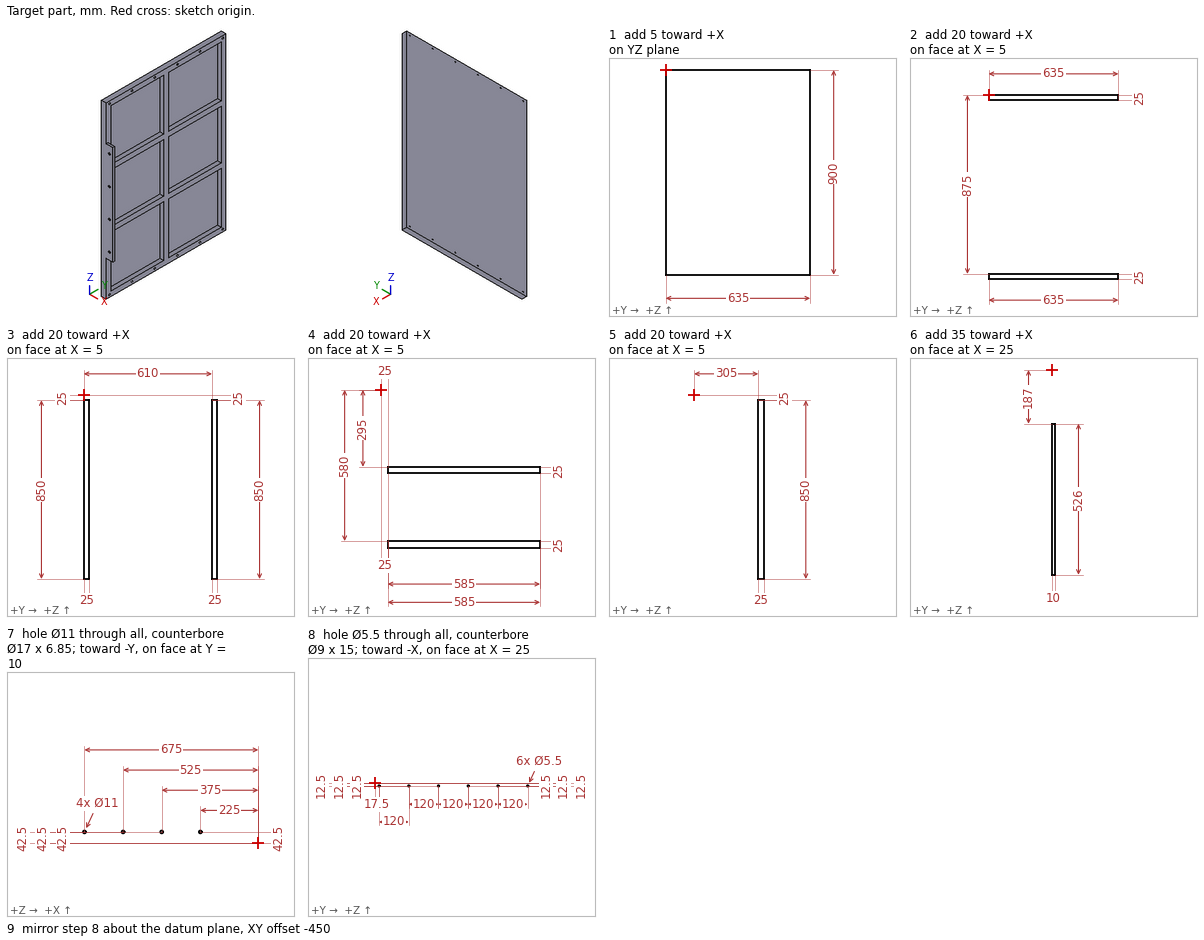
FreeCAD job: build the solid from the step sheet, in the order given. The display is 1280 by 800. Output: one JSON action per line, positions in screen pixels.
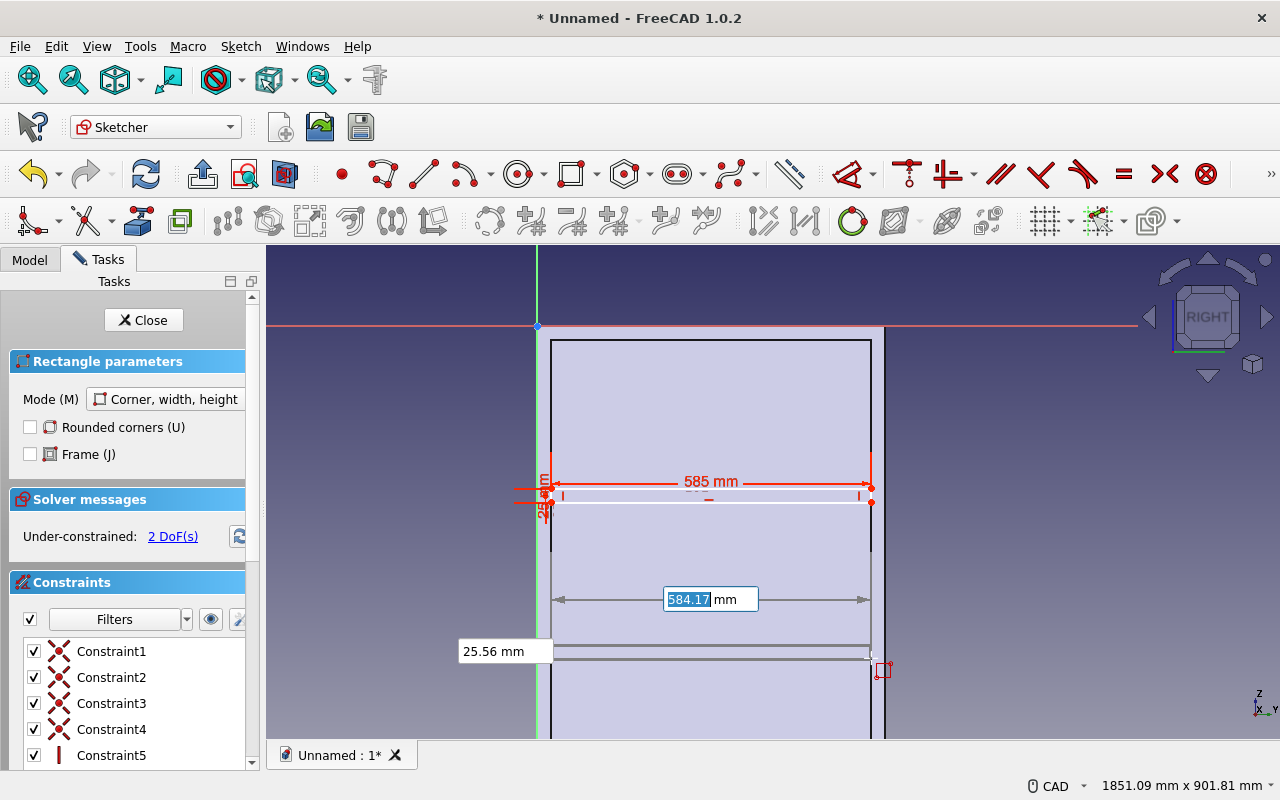
{"action": "type", "text": "585"}
{"action": "key", "text": "Tab"}
{"action": "type", "text": "25"}
{"action": "key", "text": "Return"}
{"action": "key", "text": "Escape"}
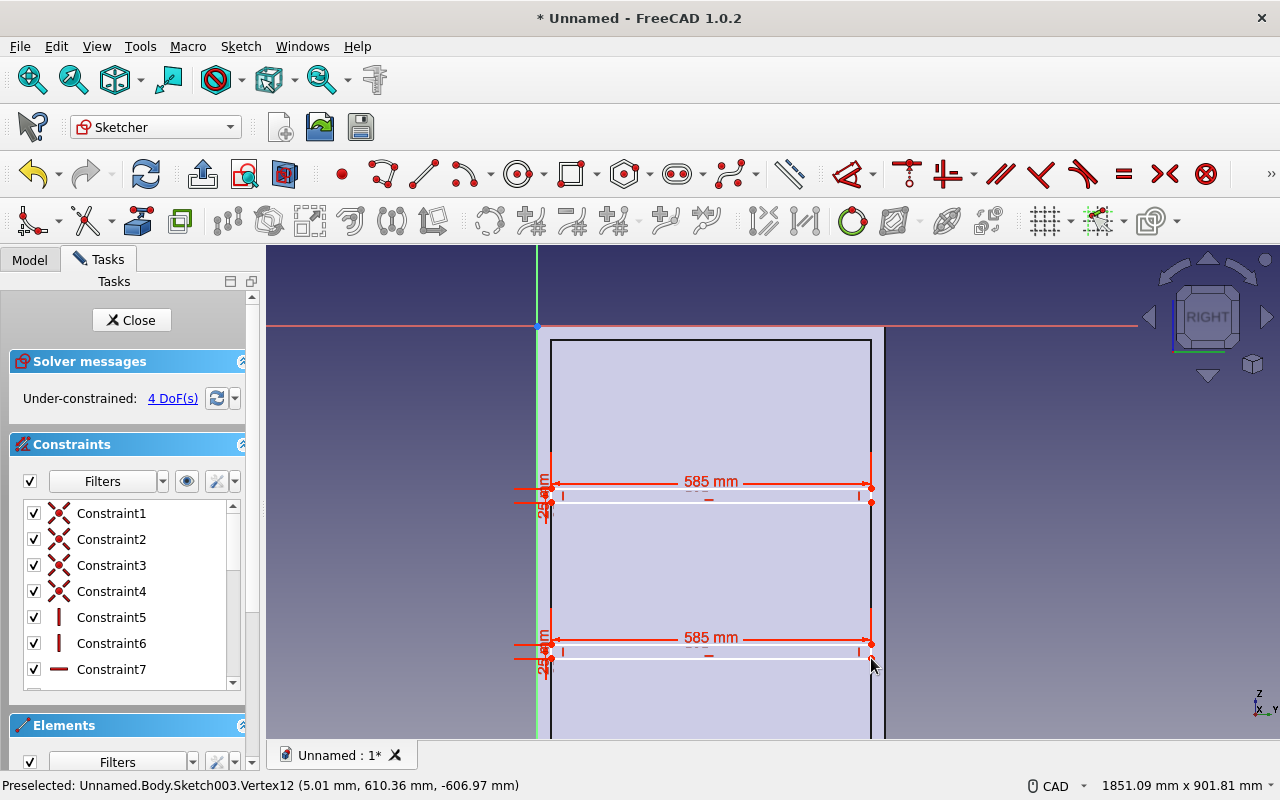
{"action": "key", "text": "d"}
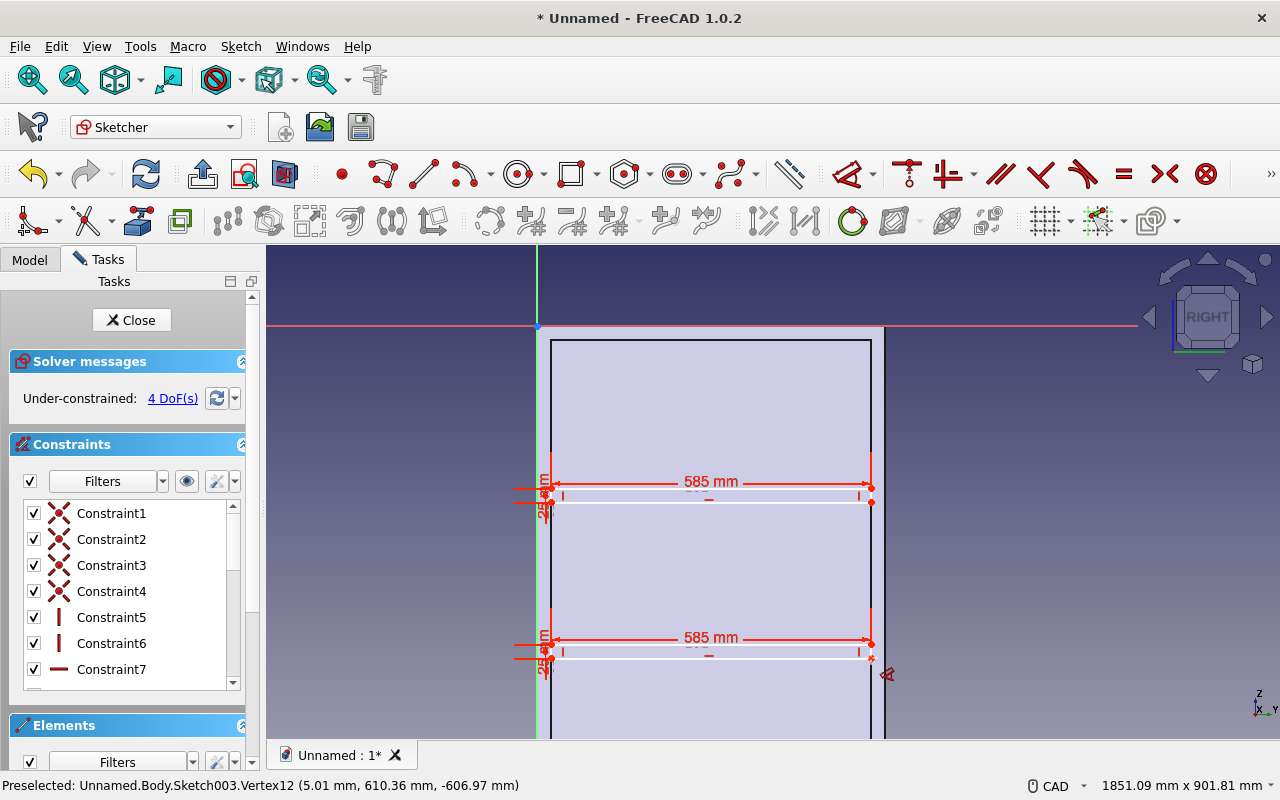
{"action": "scroll", "coordinate": [551, 489], "scroll_direction": "up", "scroll_amount": 6}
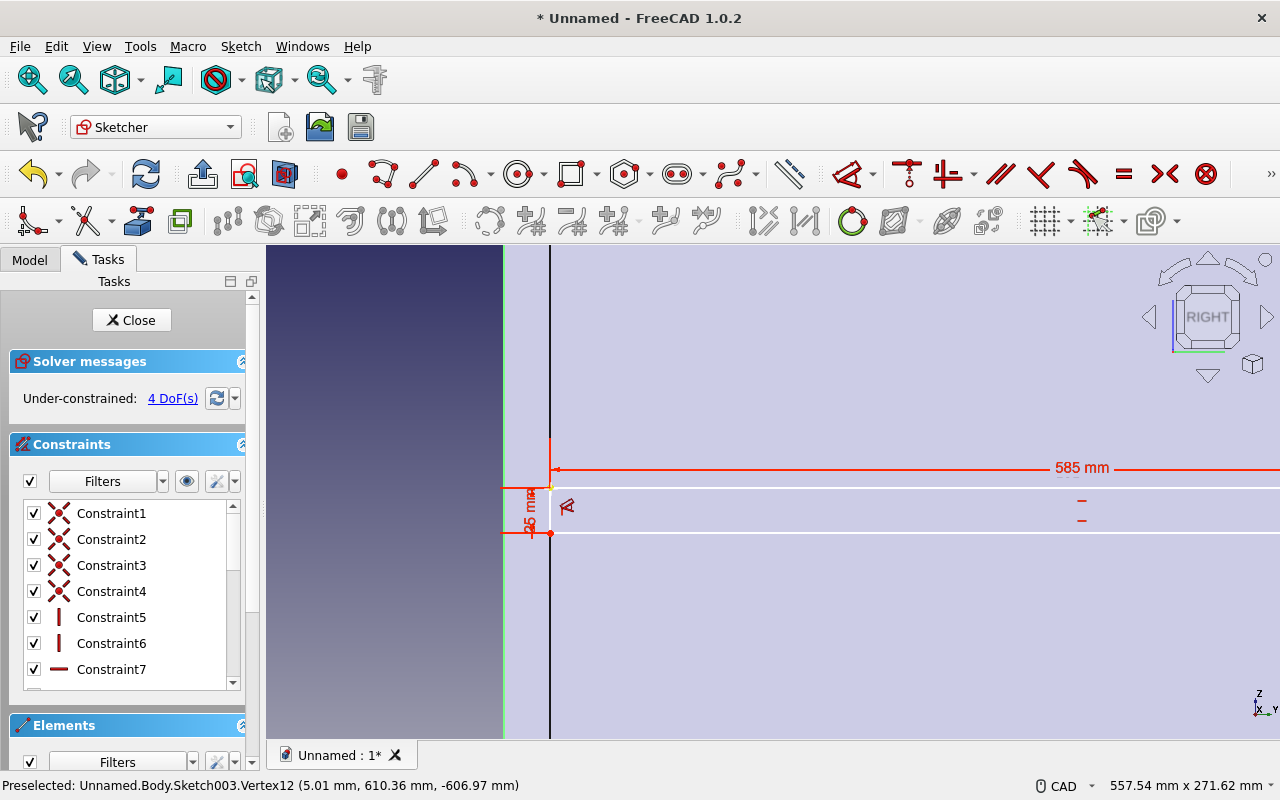
{"action": "left_click", "coordinate": [550, 488]}
{"action": "left_click", "coordinate": [527, 522]}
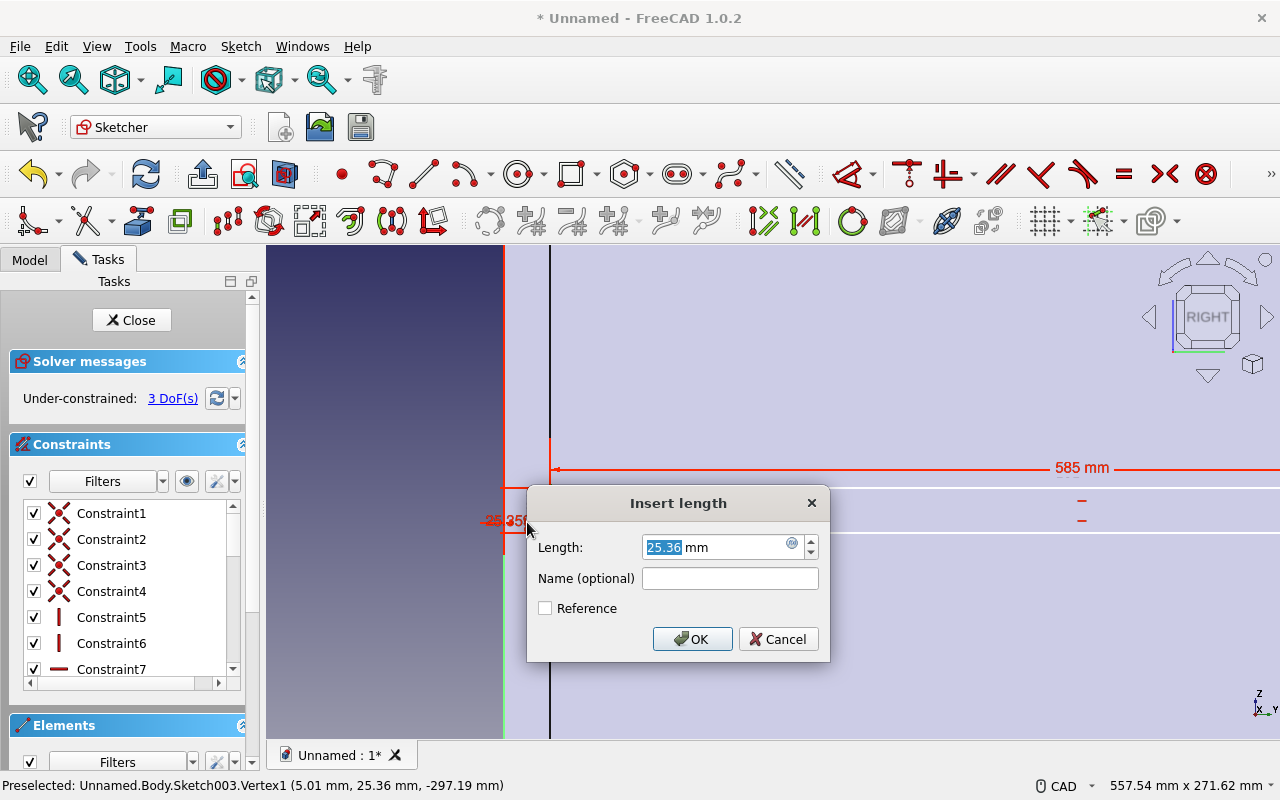
{"action": "type", "text": "25"}
{"action": "key", "text": "Return"}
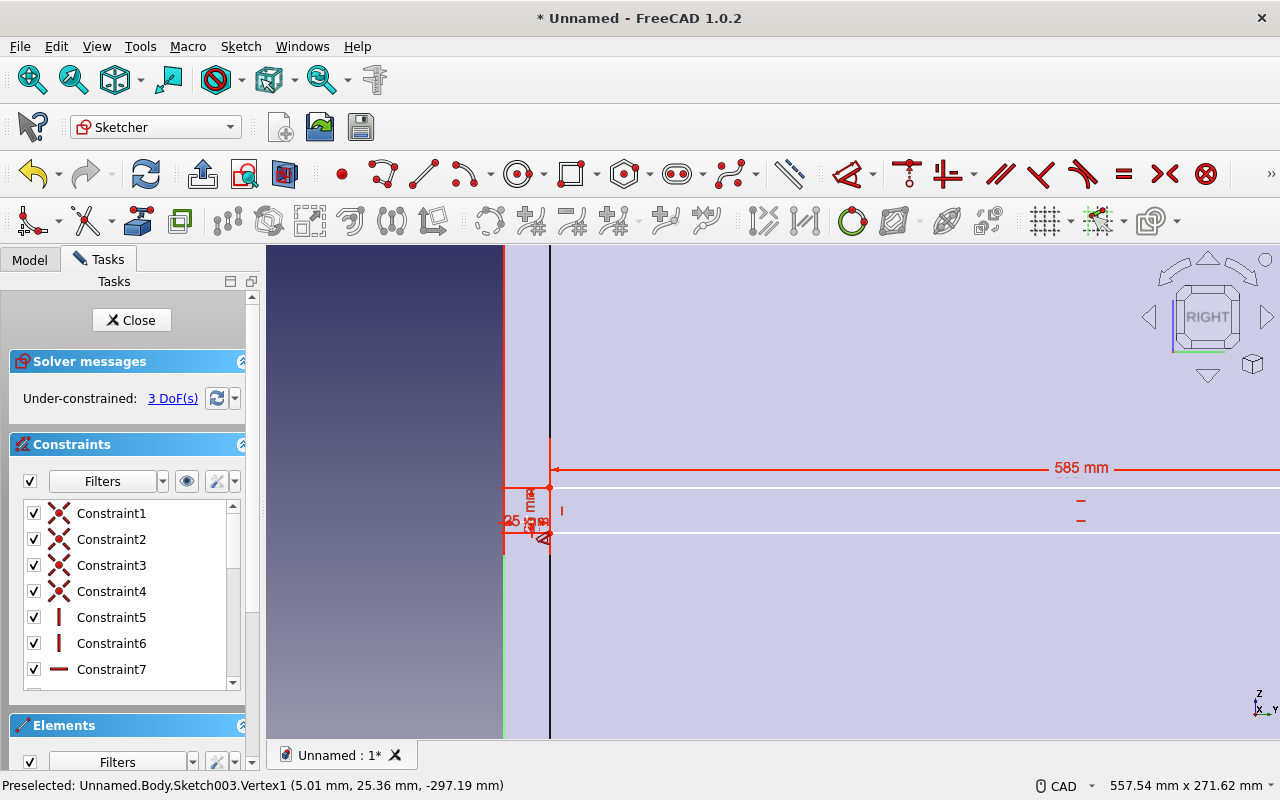
{"action": "scroll", "coordinate": [552, 490], "scroll_direction": "down", "scroll_amount": 6}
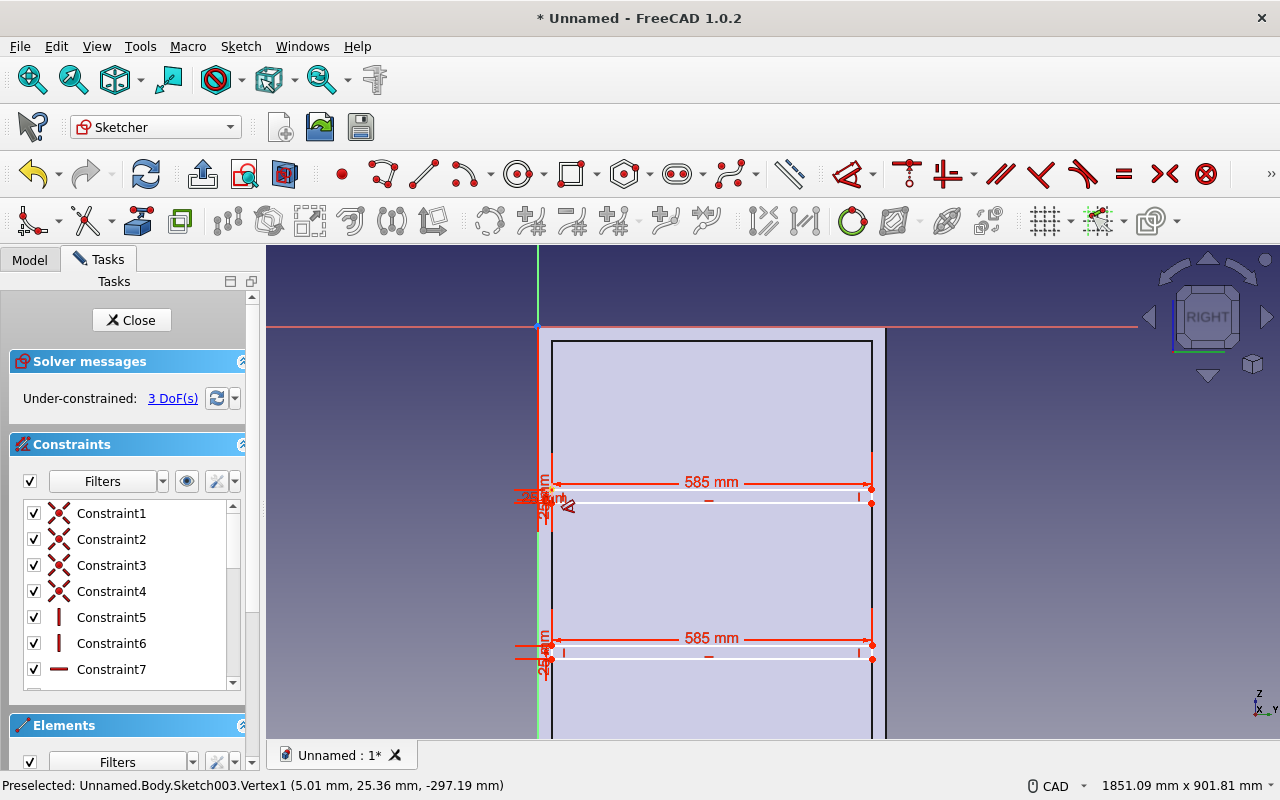
{"action": "scroll", "coordinate": [552, 646], "scroll_direction": "up", "scroll_amount": 6}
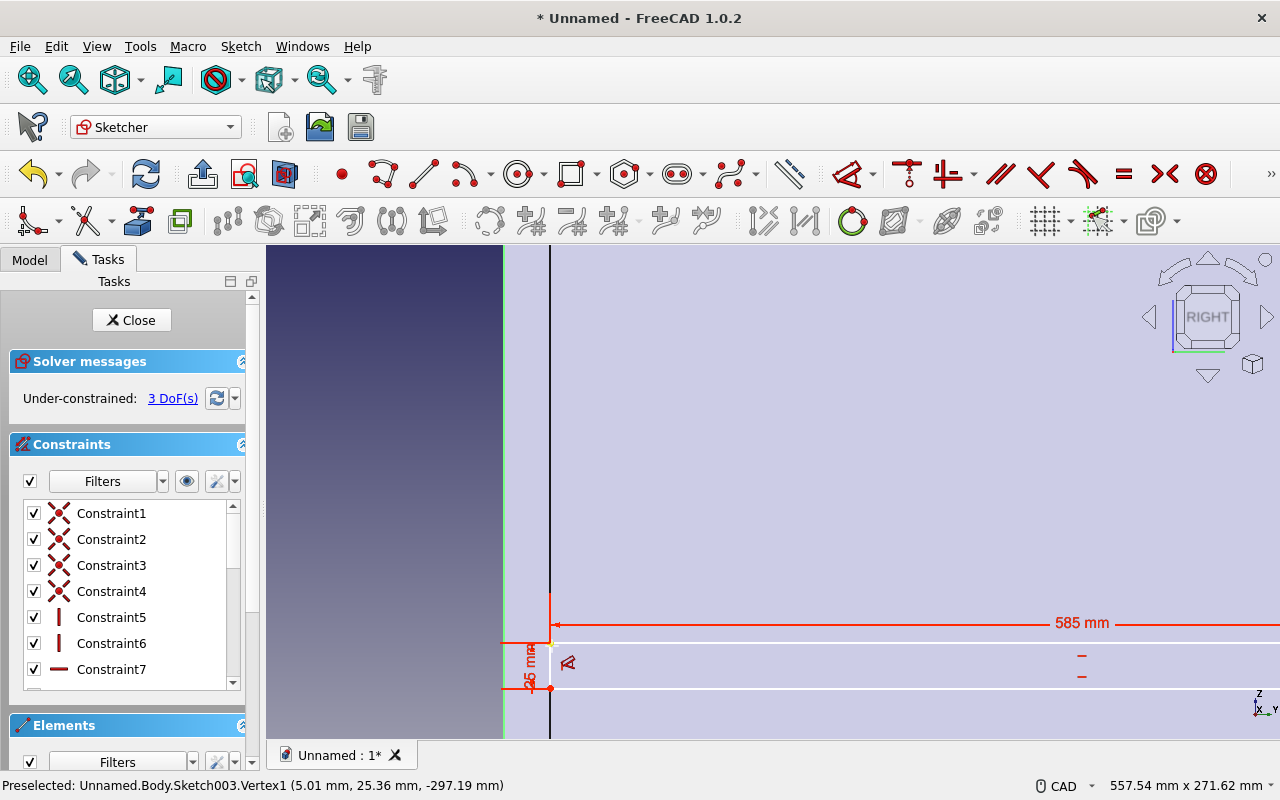
{"action": "left_click", "coordinate": [550, 643]}
{"action": "left_click", "coordinate": [527, 677]}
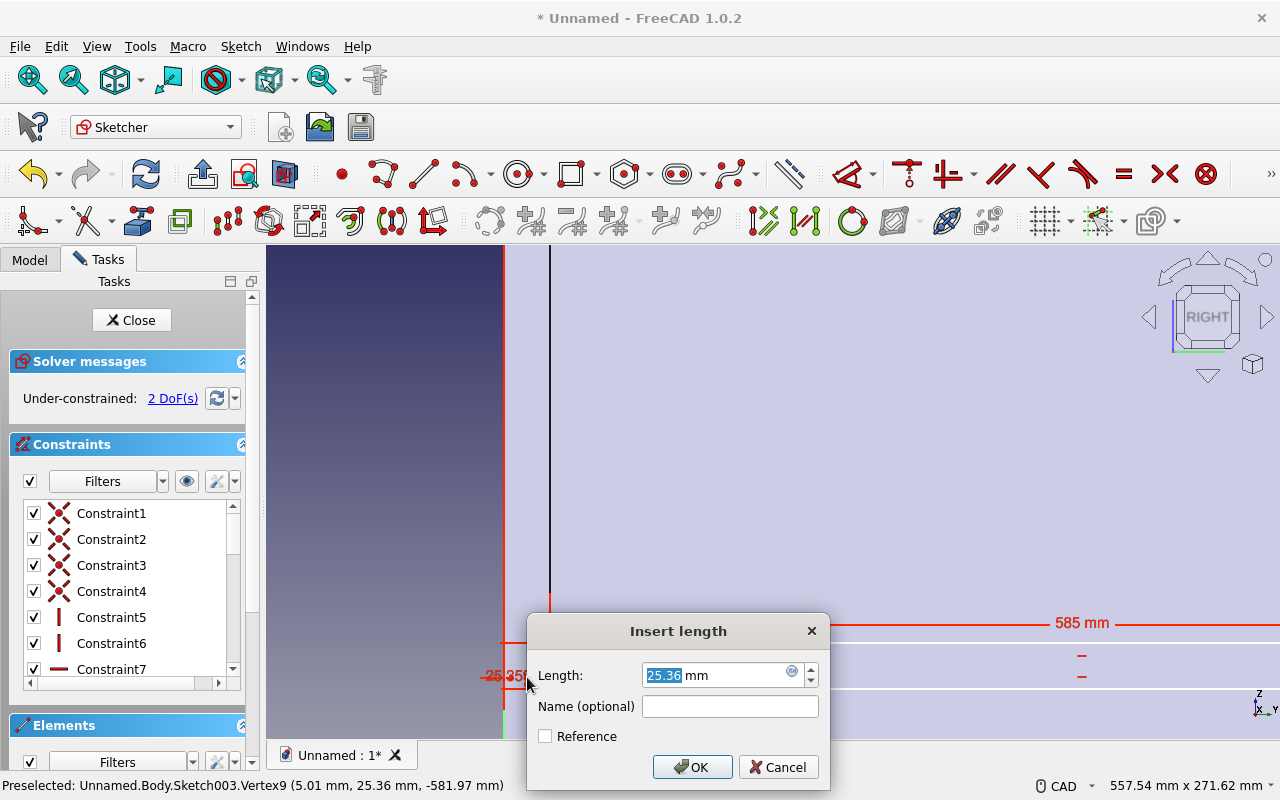
{"action": "type", "text": "25"}
{"action": "key", "text": "Return"}